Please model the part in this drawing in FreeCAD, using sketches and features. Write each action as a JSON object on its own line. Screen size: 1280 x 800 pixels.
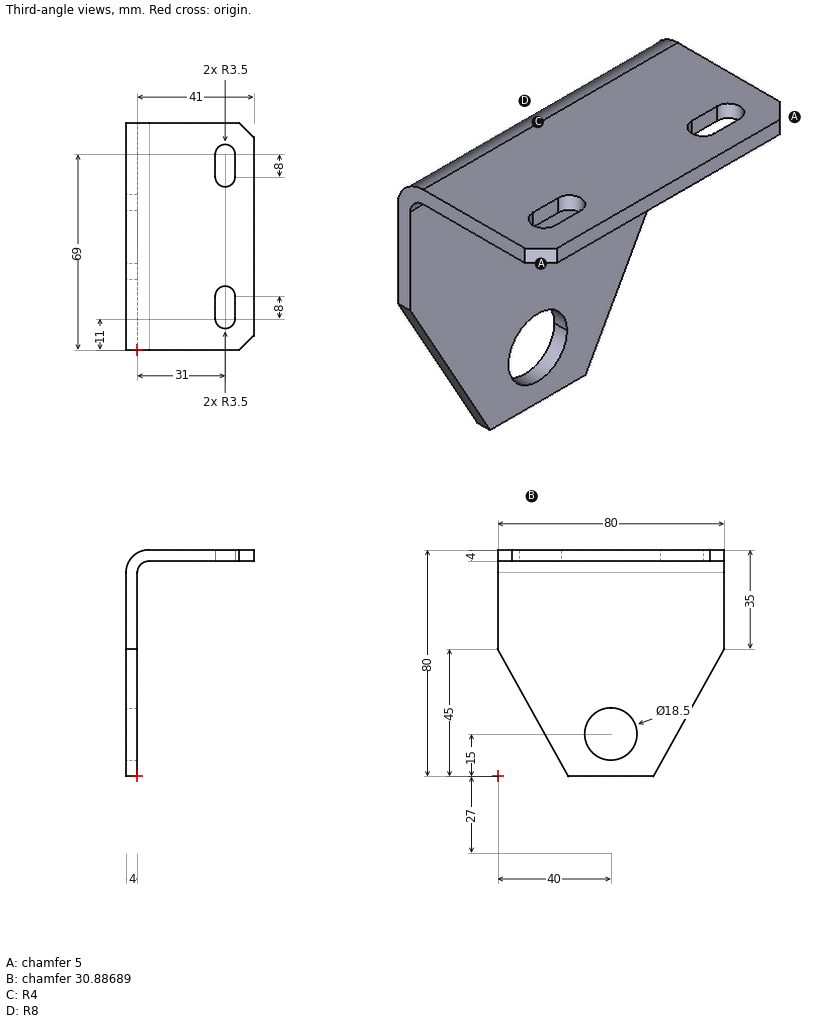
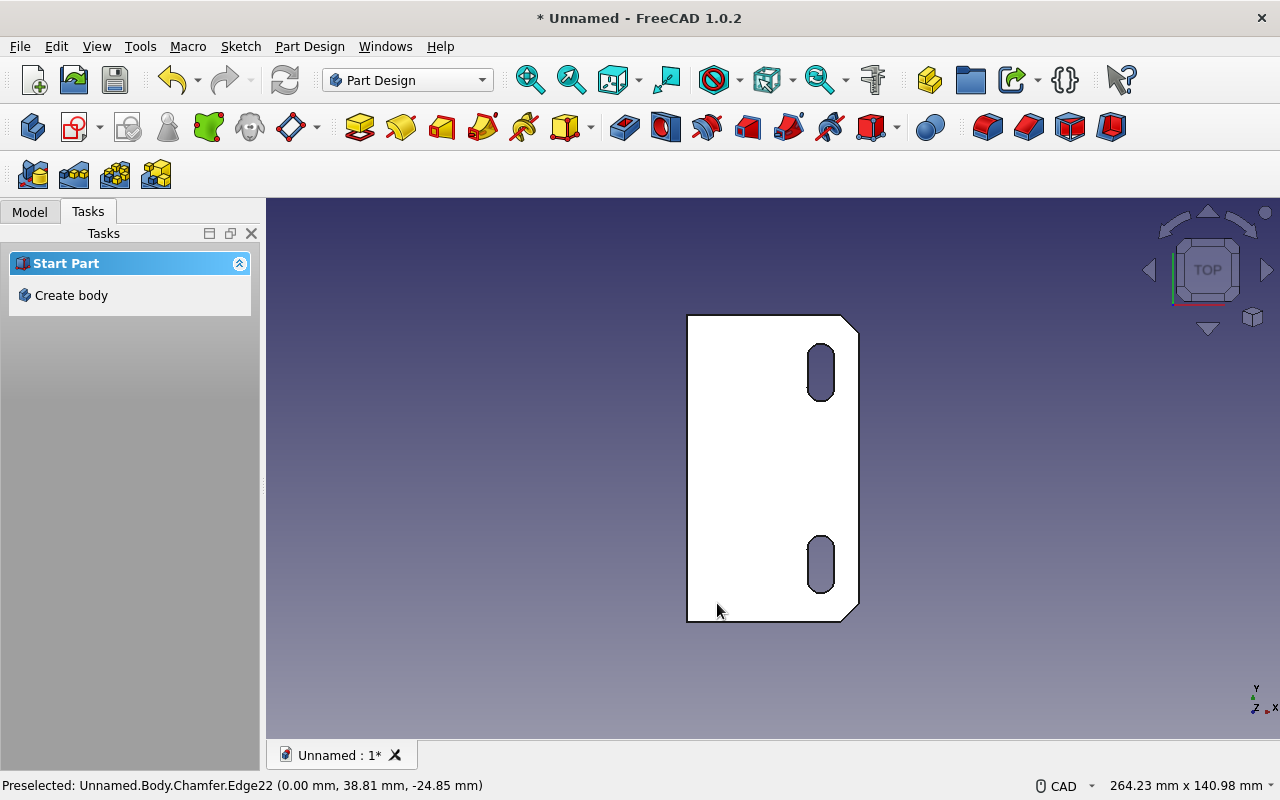
{"action": "scroll", "coordinate": [694, 467], "scroll_direction": "up", "scroll_amount": 5}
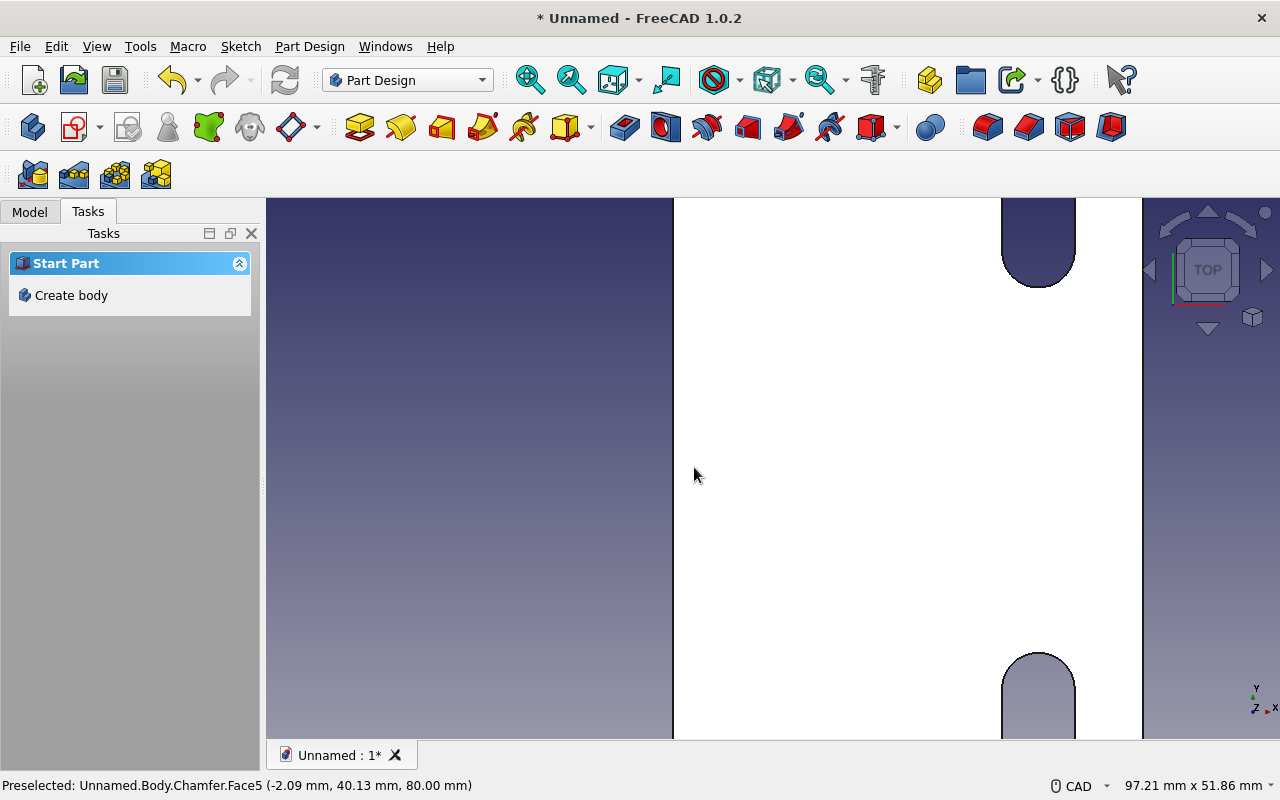
{"action": "left_click", "coordinate": [531, 80]}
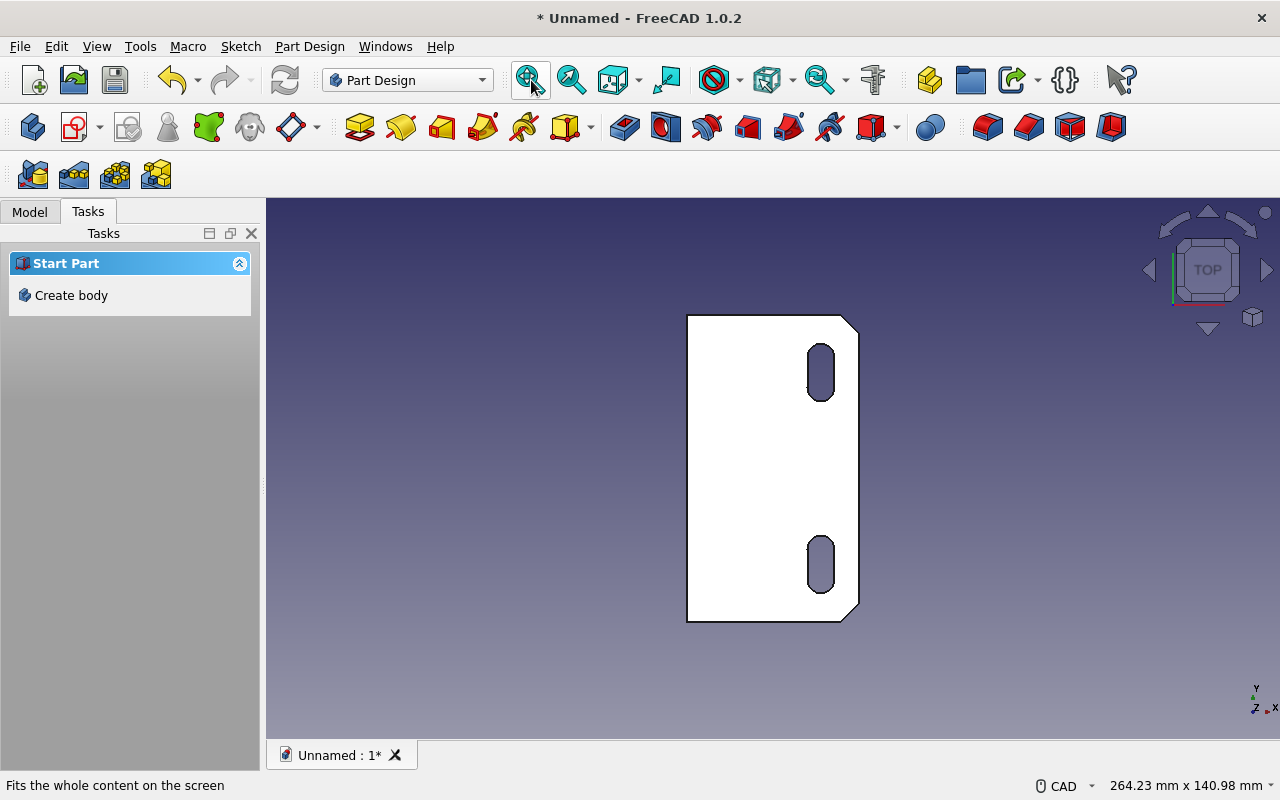
{"action": "key", "text": "1"}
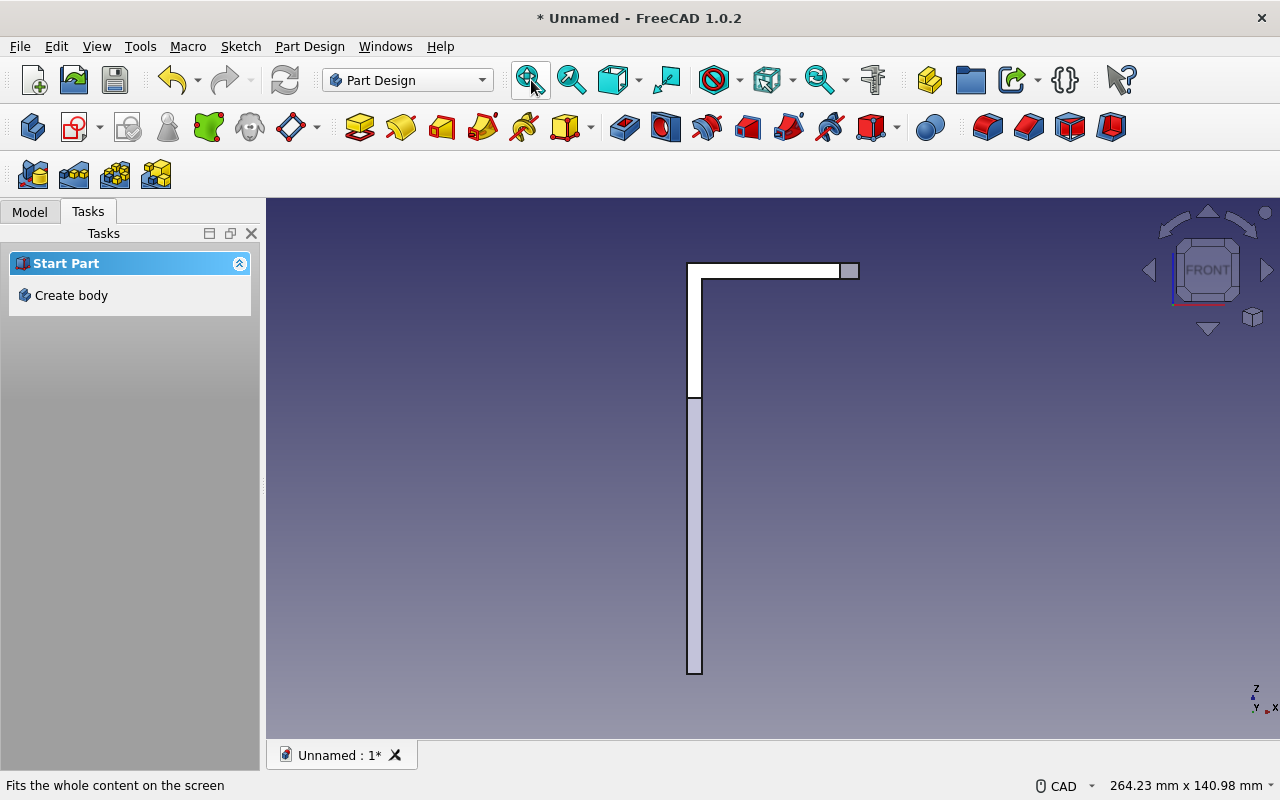
{"action": "scroll", "coordinate": [694, 673], "scroll_direction": "up", "scroll_amount": 5}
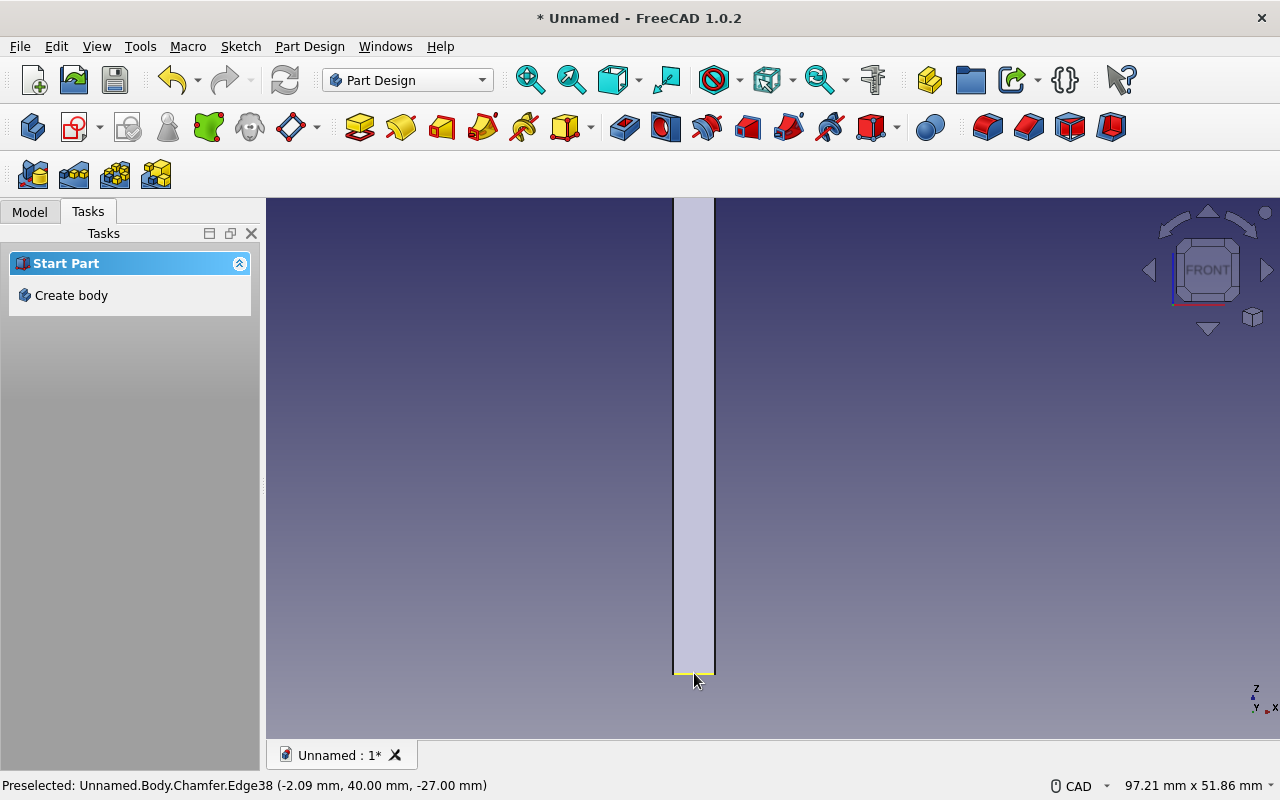
{"action": "left_click", "coordinate": [531, 80]}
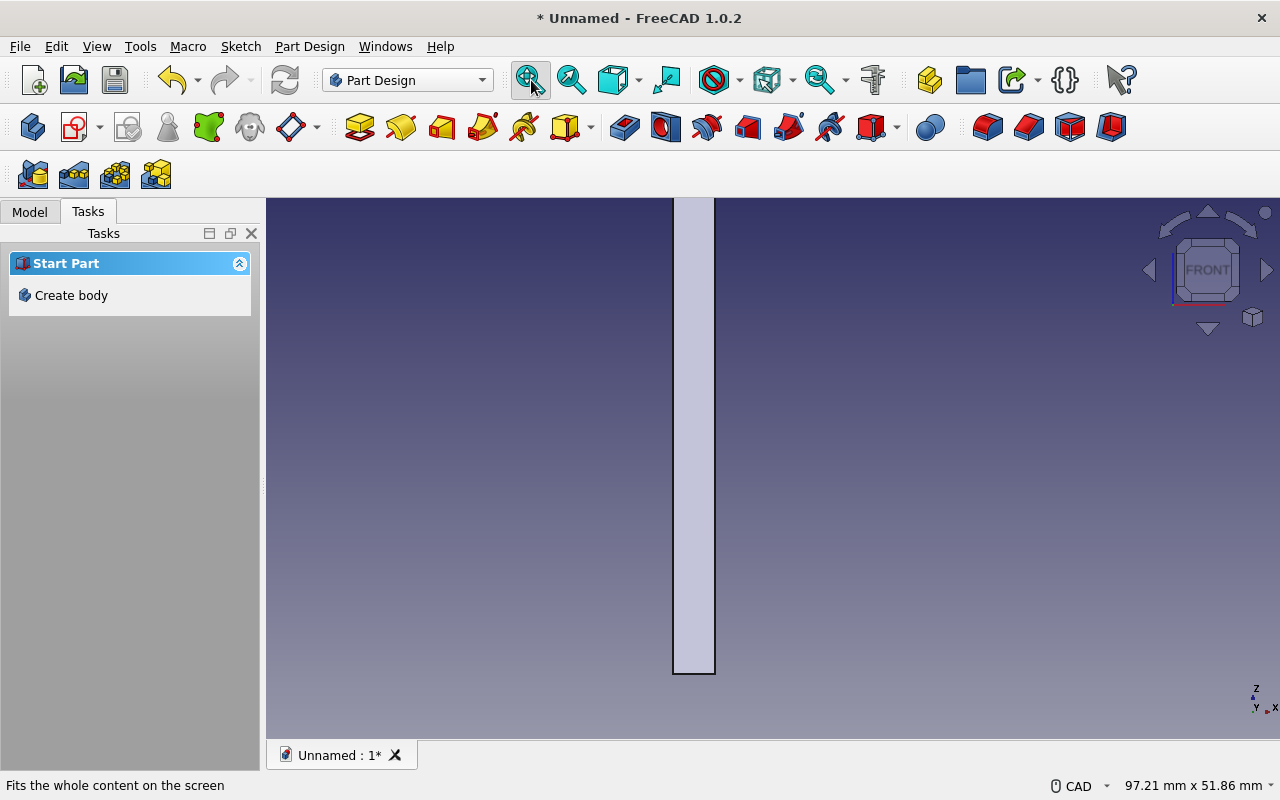
{"action": "key", "text": "3"}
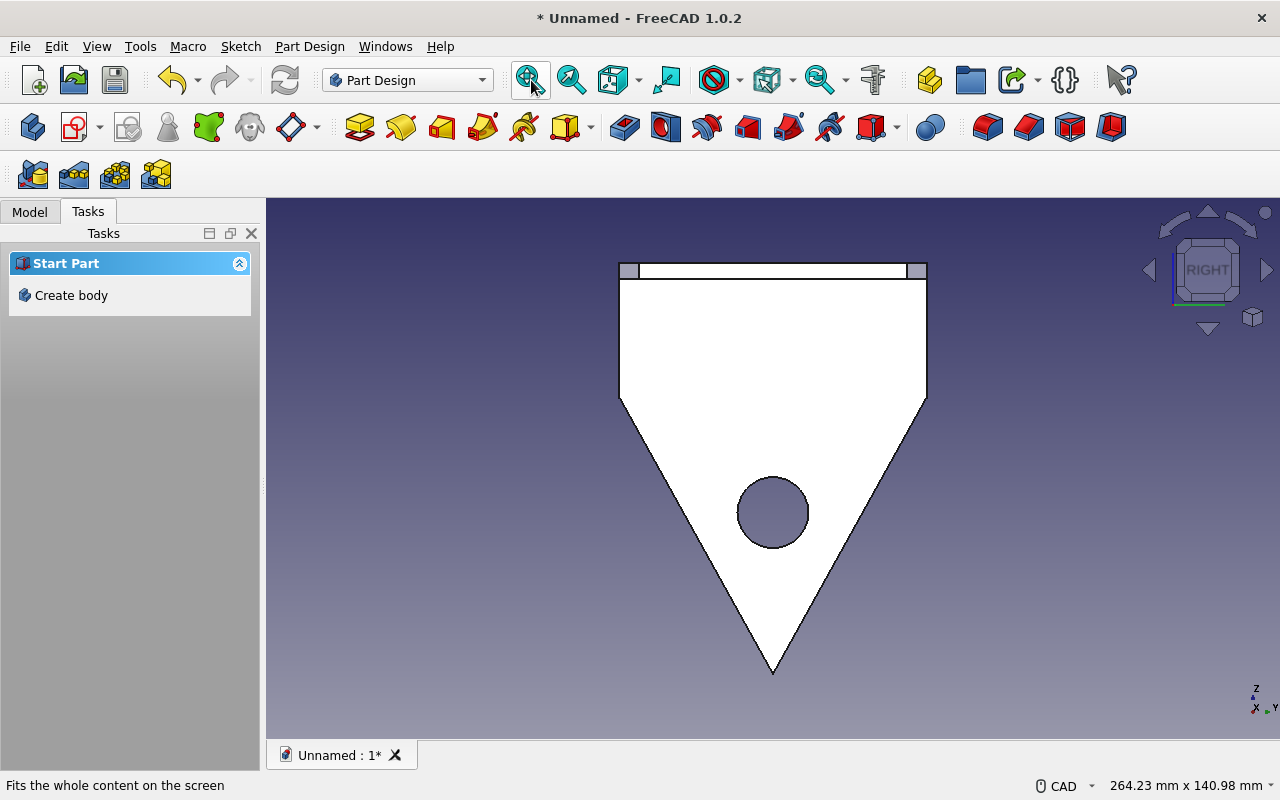
{"action": "scroll", "coordinate": [773, 673], "scroll_direction": "up", "scroll_amount": 5}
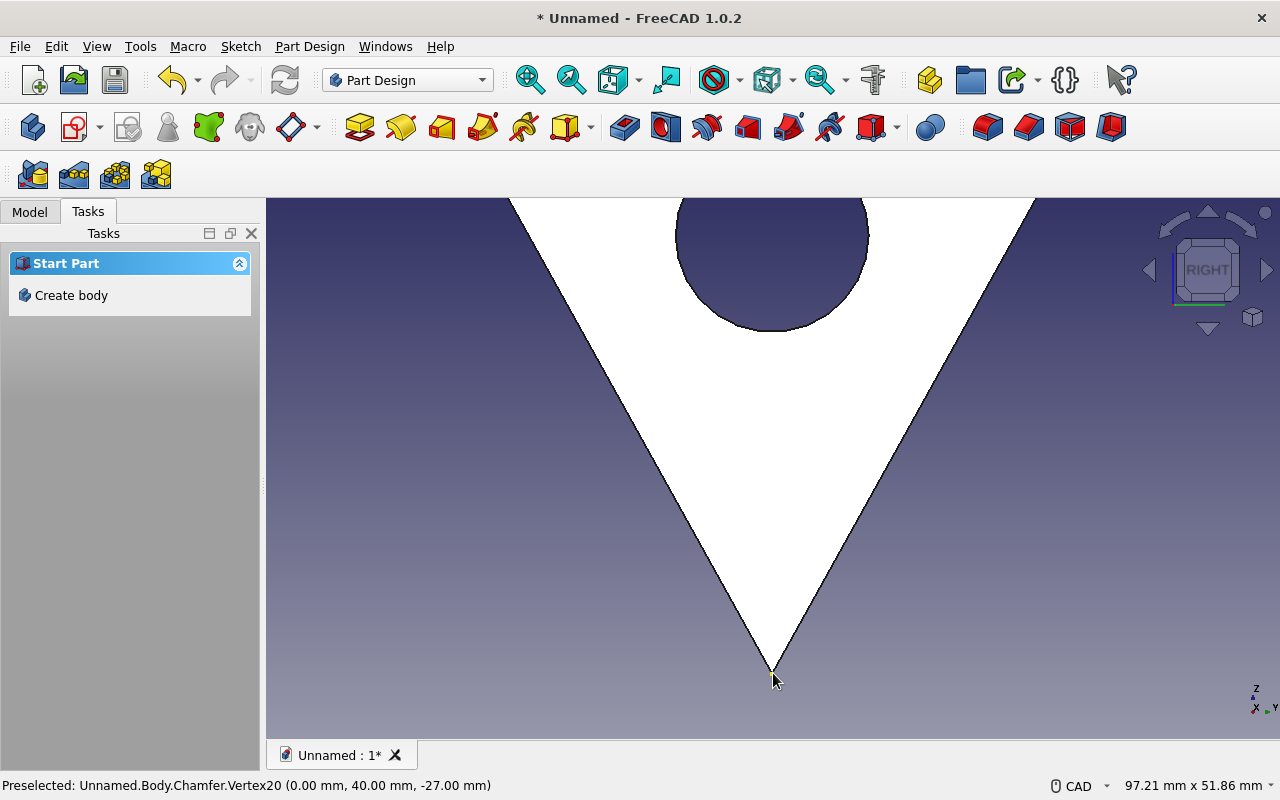
{"action": "left_click", "coordinate": [531, 80]}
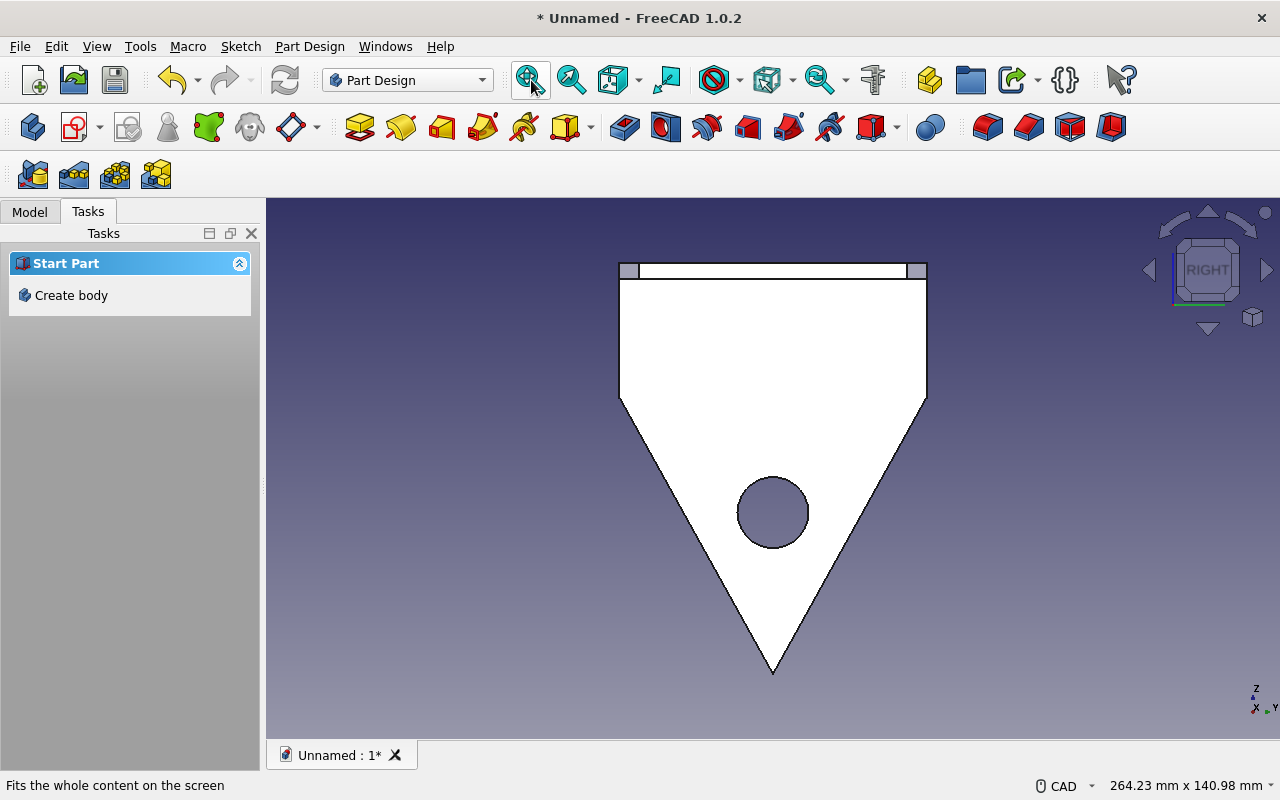
{"action": "key", "text": "5"}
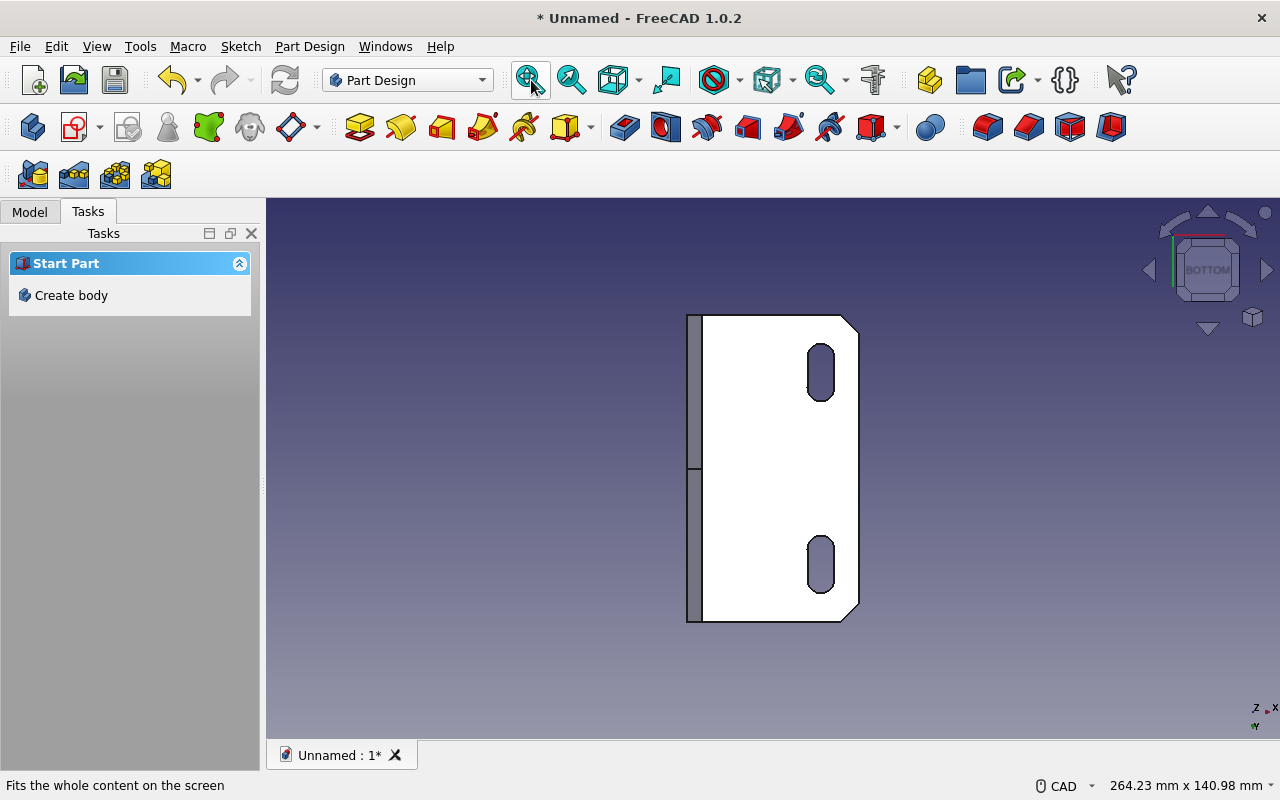
{"action": "left_click", "coordinate": [694, 467]}